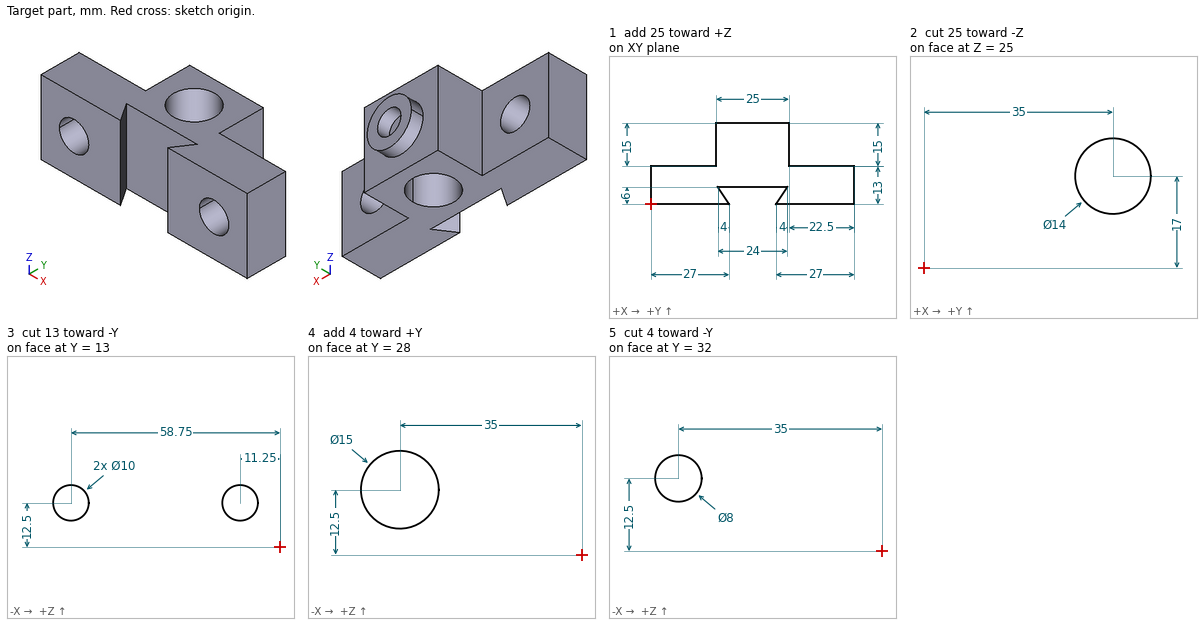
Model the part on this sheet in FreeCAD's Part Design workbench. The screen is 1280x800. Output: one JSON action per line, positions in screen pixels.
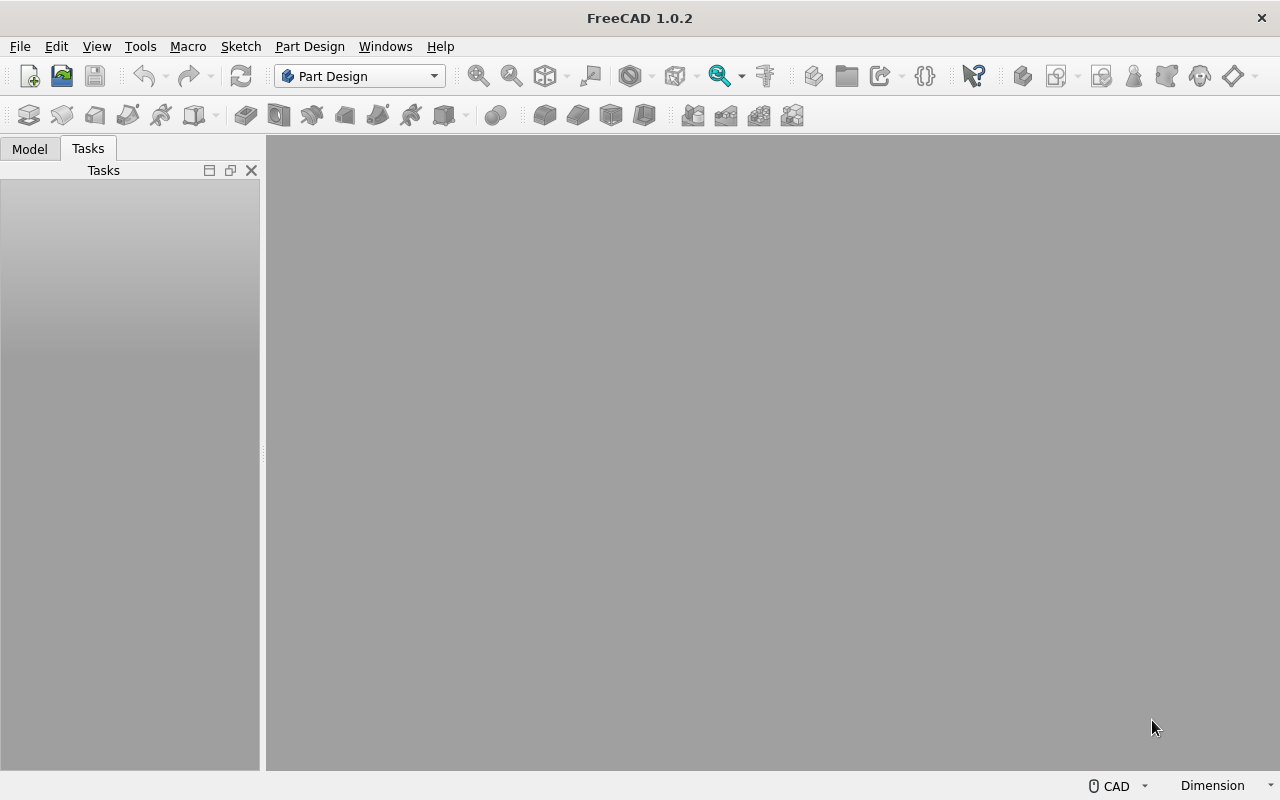
{"action": "left_click", "coordinate": [29, 76]}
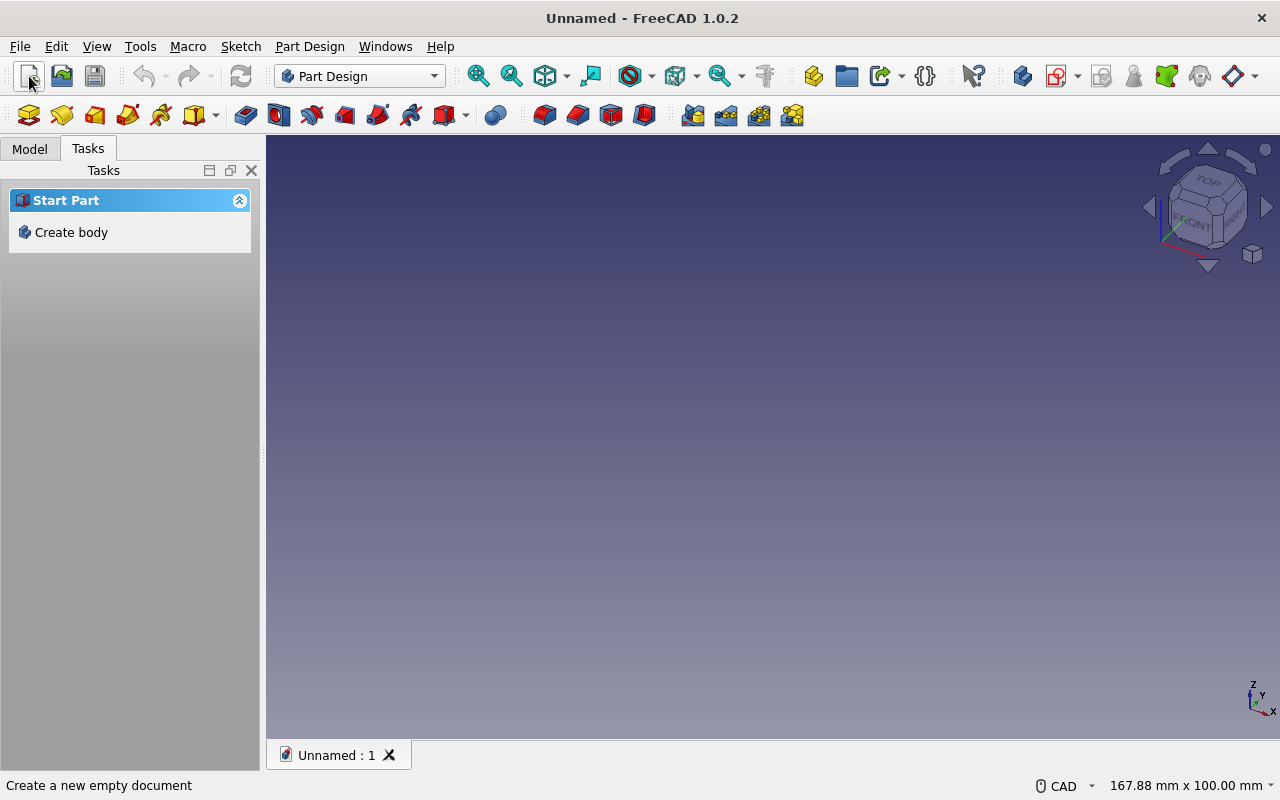
{"action": "left_click", "coordinate": [1056, 76]}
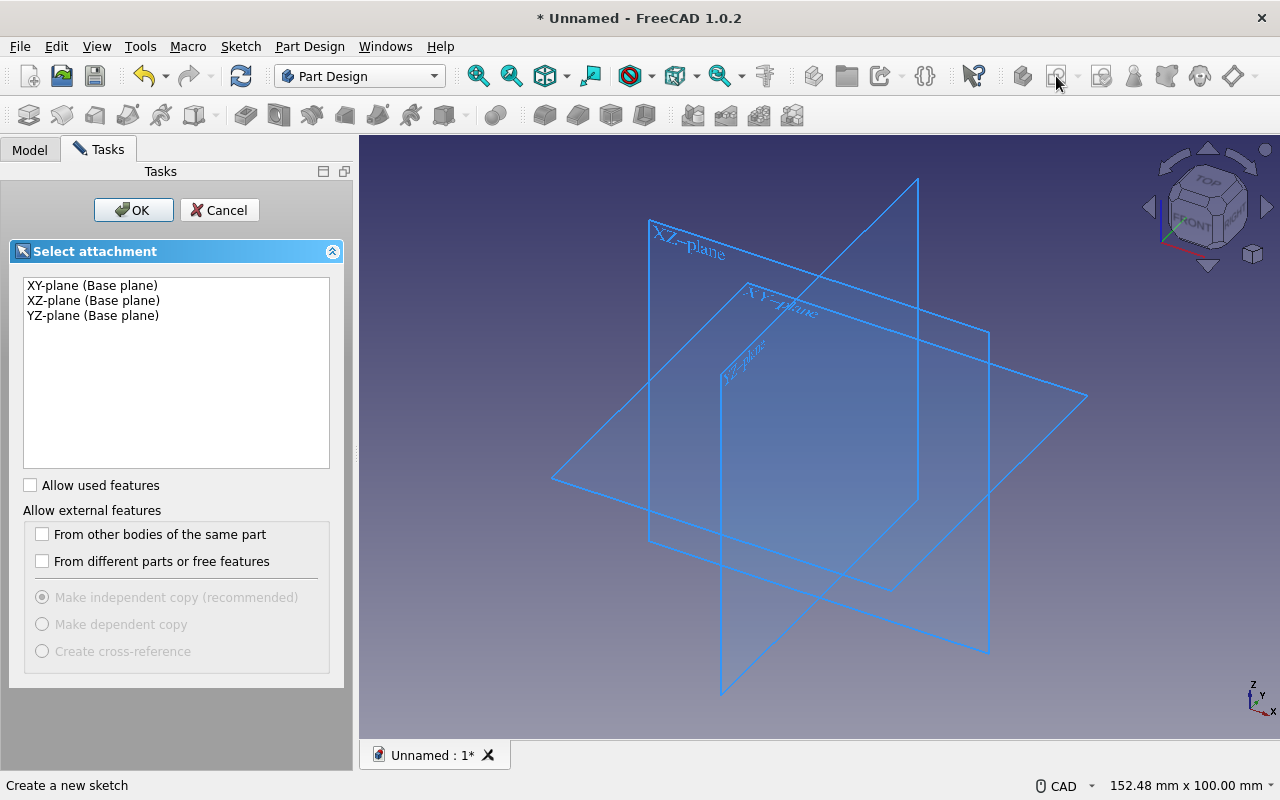
{"action": "left_click", "coordinate": [84, 286]}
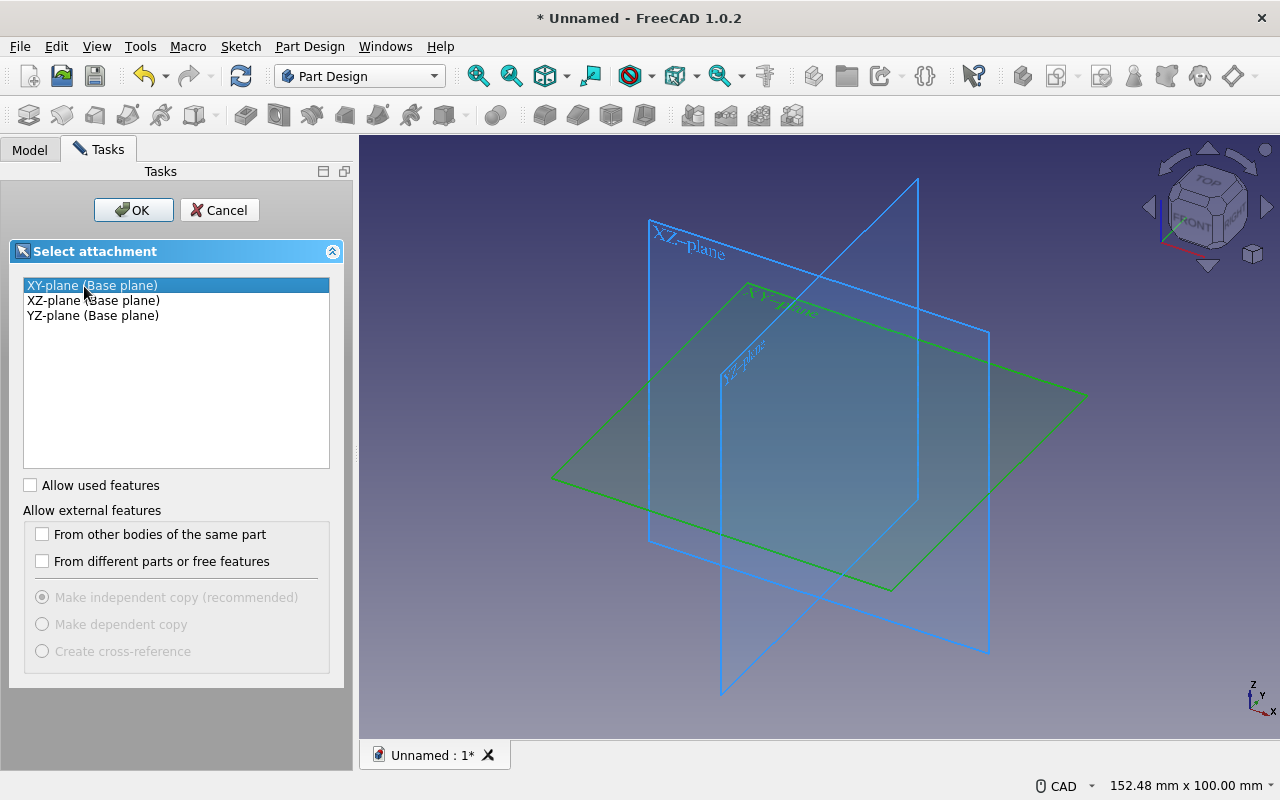
{"action": "left_click", "coordinate": [134, 210]}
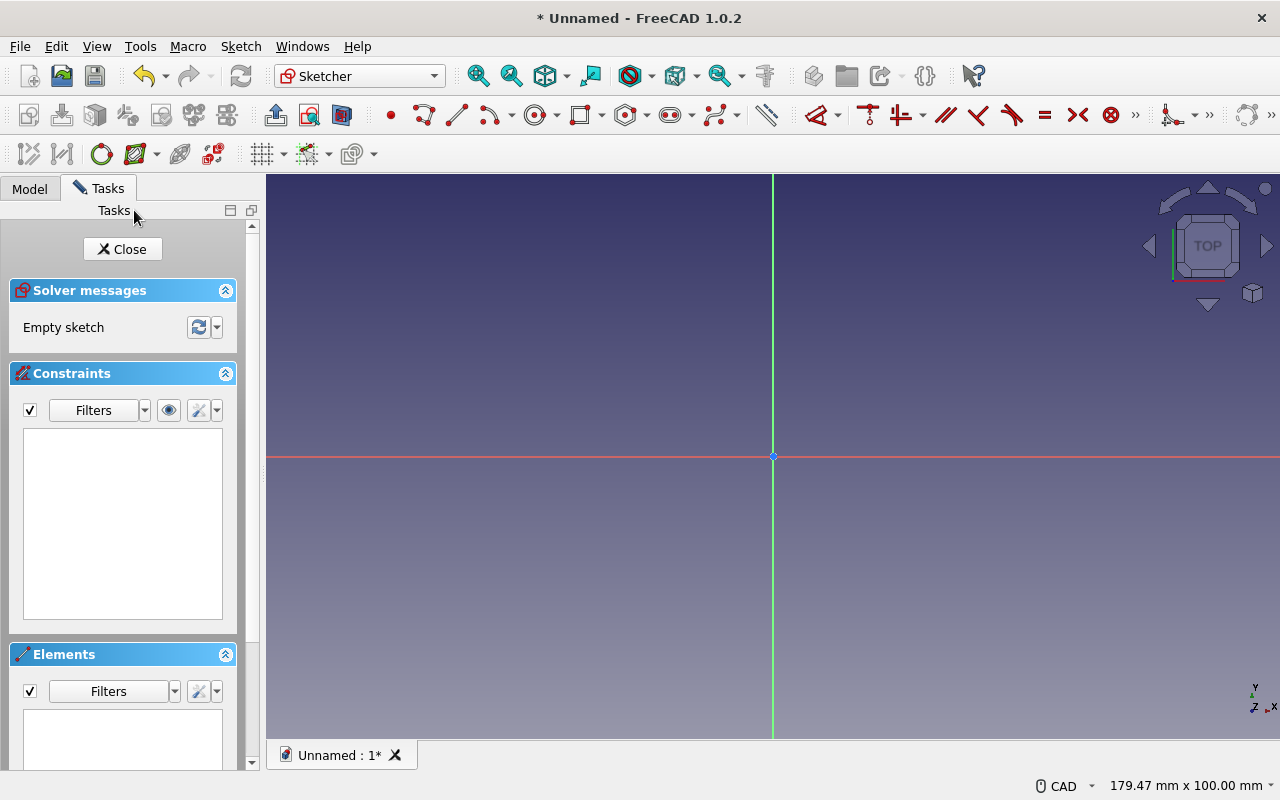
{"action": "scroll", "coordinate": [294, 711], "scroll_direction": "down", "scroll_amount": 1}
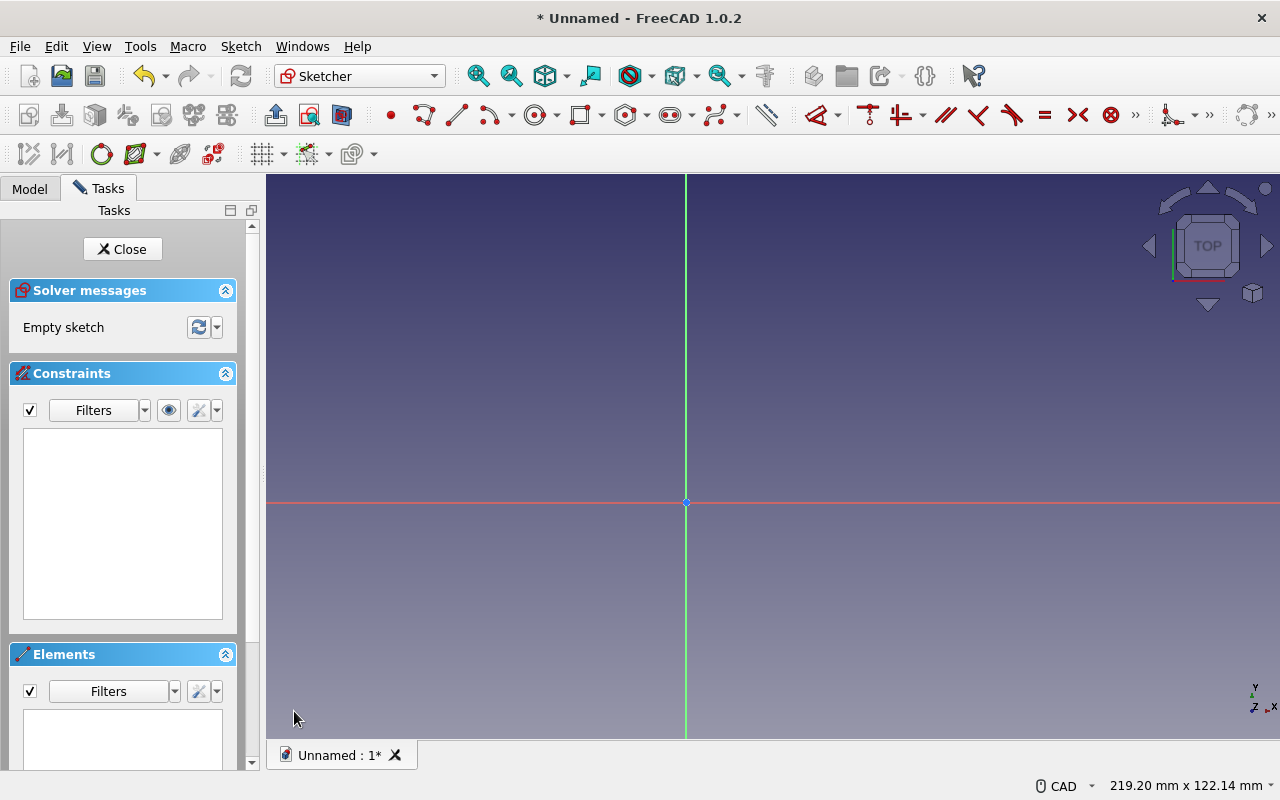
{"action": "scroll", "coordinate": [1023, 416], "scroll_direction": "up", "scroll_amount": 3}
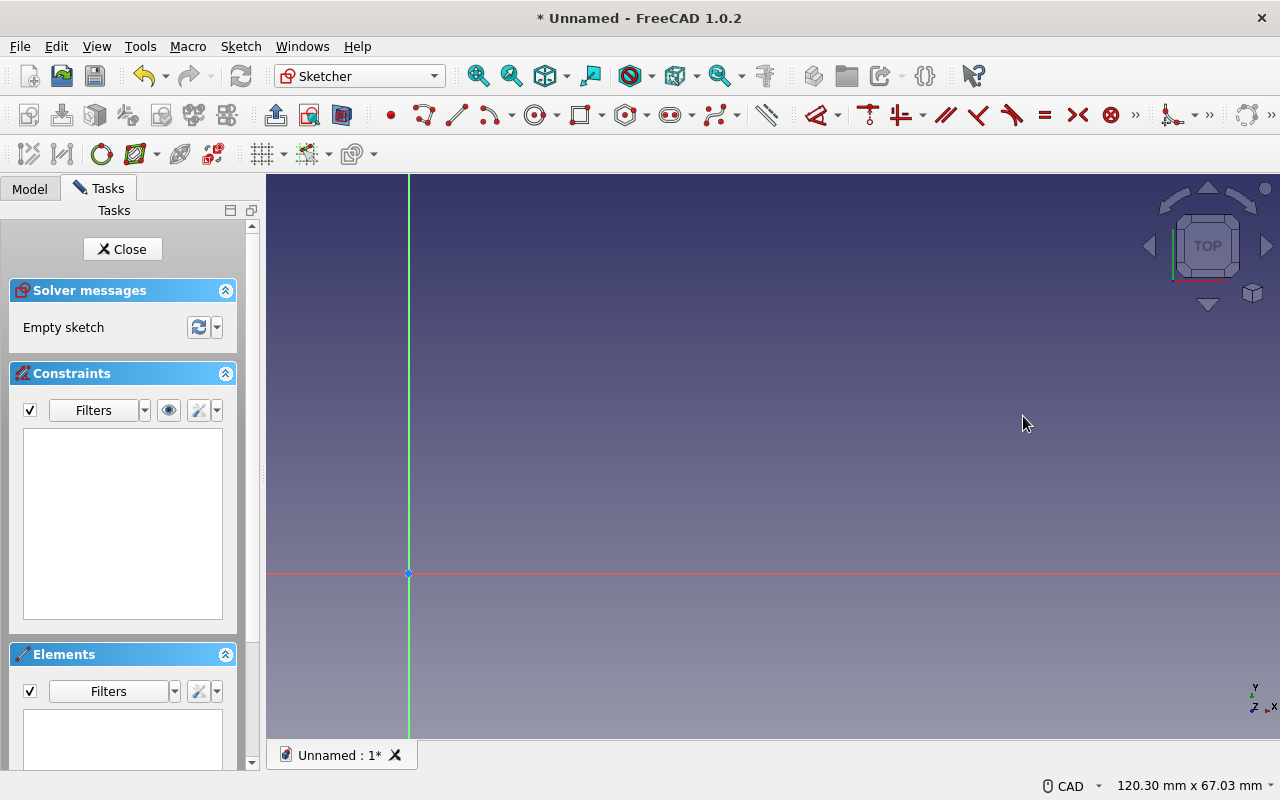
{"action": "left_click", "coordinate": [424, 116]}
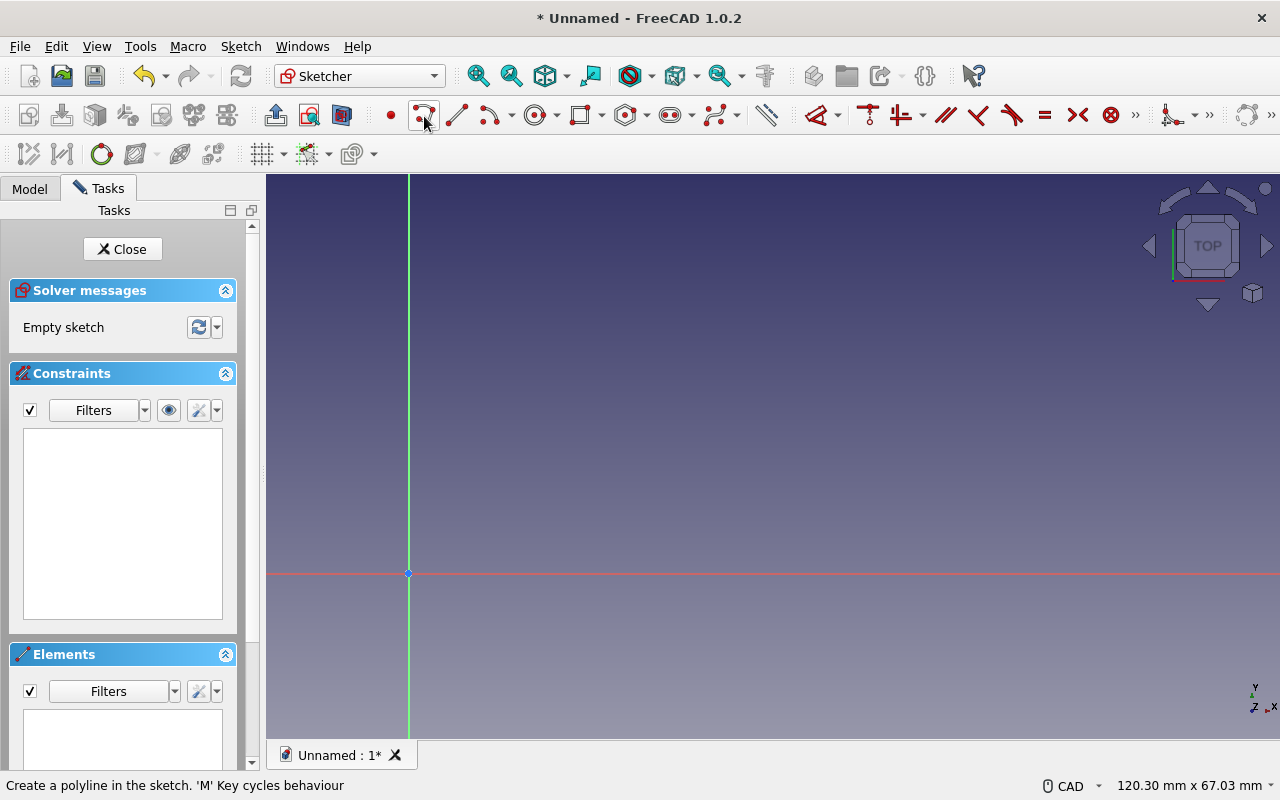
{"action": "left_click", "coordinate": [409, 574]}
{"action": "left_click", "coordinate": [636, 565]}
{"action": "left_click", "coordinate": [603, 523]}
{"action": "left_click", "coordinate": [805, 523]}
{"action": "left_click", "coordinate": [771, 574]}
{"action": "left_click", "coordinate": [999, 565]}
{"action": "left_click", "coordinate": [999, 464]}
{"action": "left_click", "coordinate": [809, 464]}
{"action": "left_click", "coordinate": [809, 338]}
{"action": "left_click", "coordinate": [598, 338]}
{"action": "left_click", "coordinate": [598, 464]}
{"action": "left_click", "coordinate": [418, 464]}
{"action": "left_click", "coordinate": [409, 574]}
{"action": "key", "text": "Escape"}
{"action": "key", "text": "Escape"}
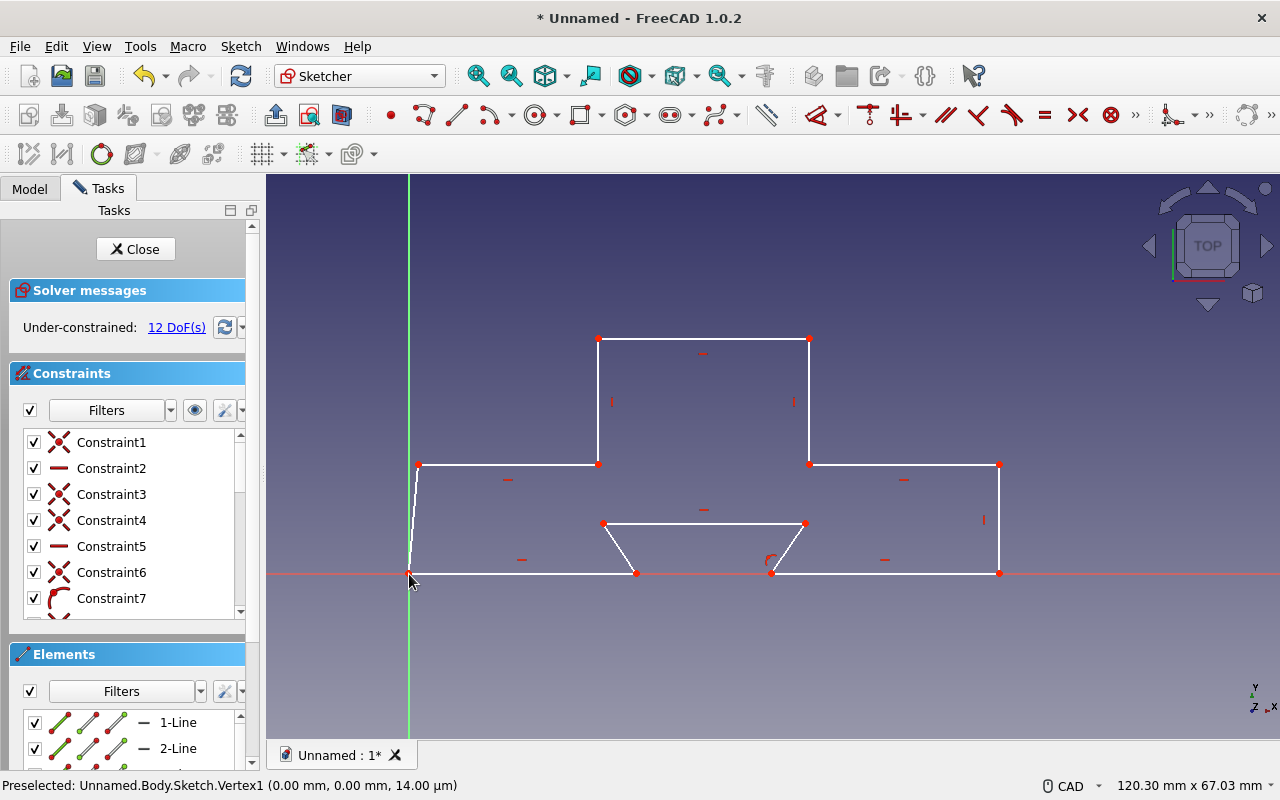
{"action": "left_click", "coordinate": [411, 541]}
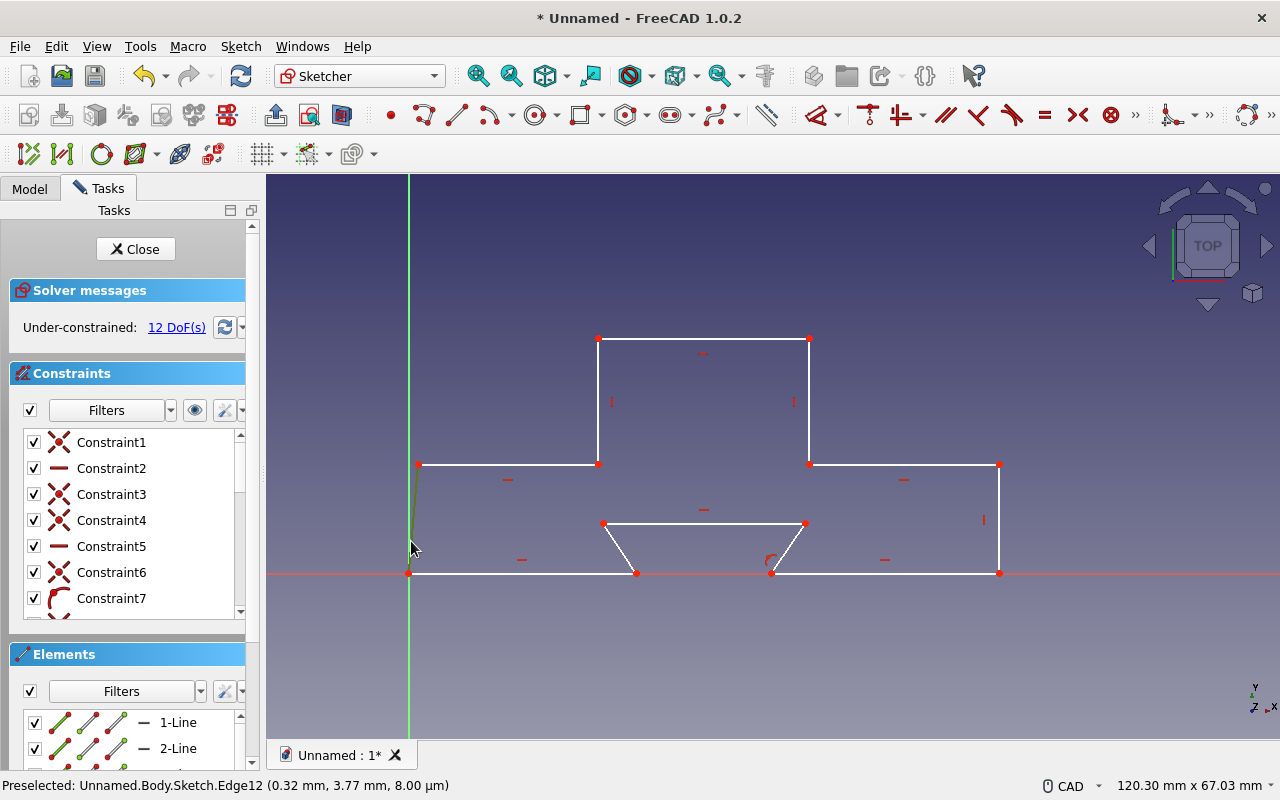
{"action": "key", "text": "v"}